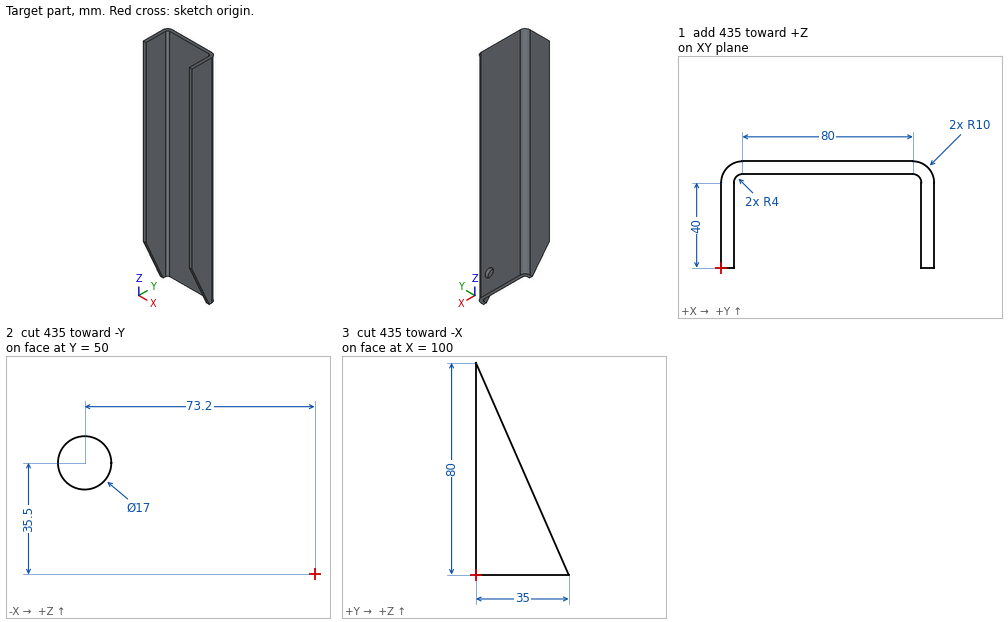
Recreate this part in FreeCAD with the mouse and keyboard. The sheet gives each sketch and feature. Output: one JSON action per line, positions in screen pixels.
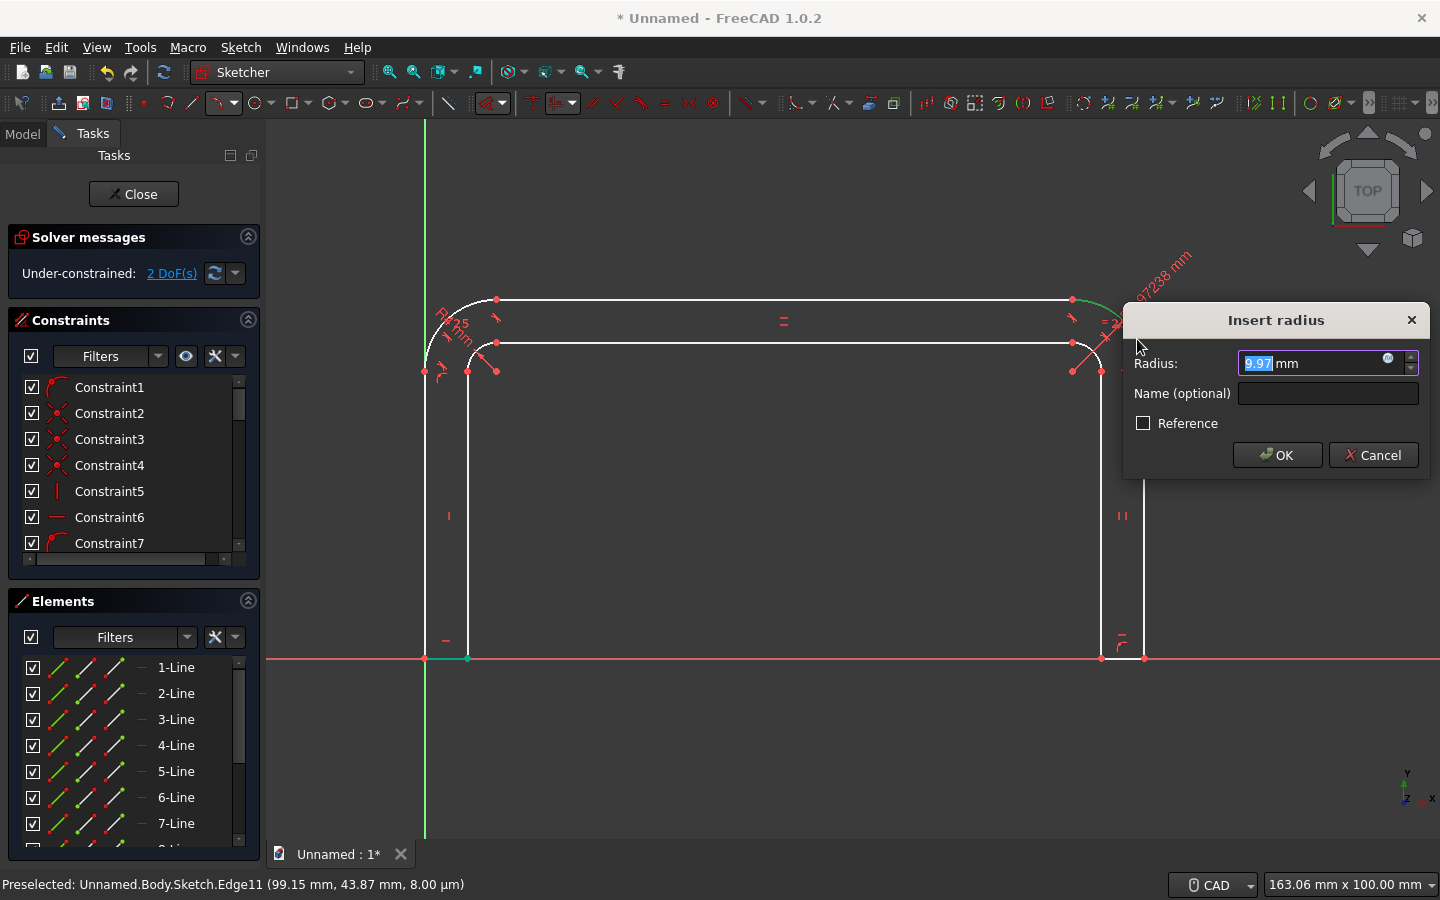
{"action": "type", "text": "10"}
{"action": "key", "text": "Return"}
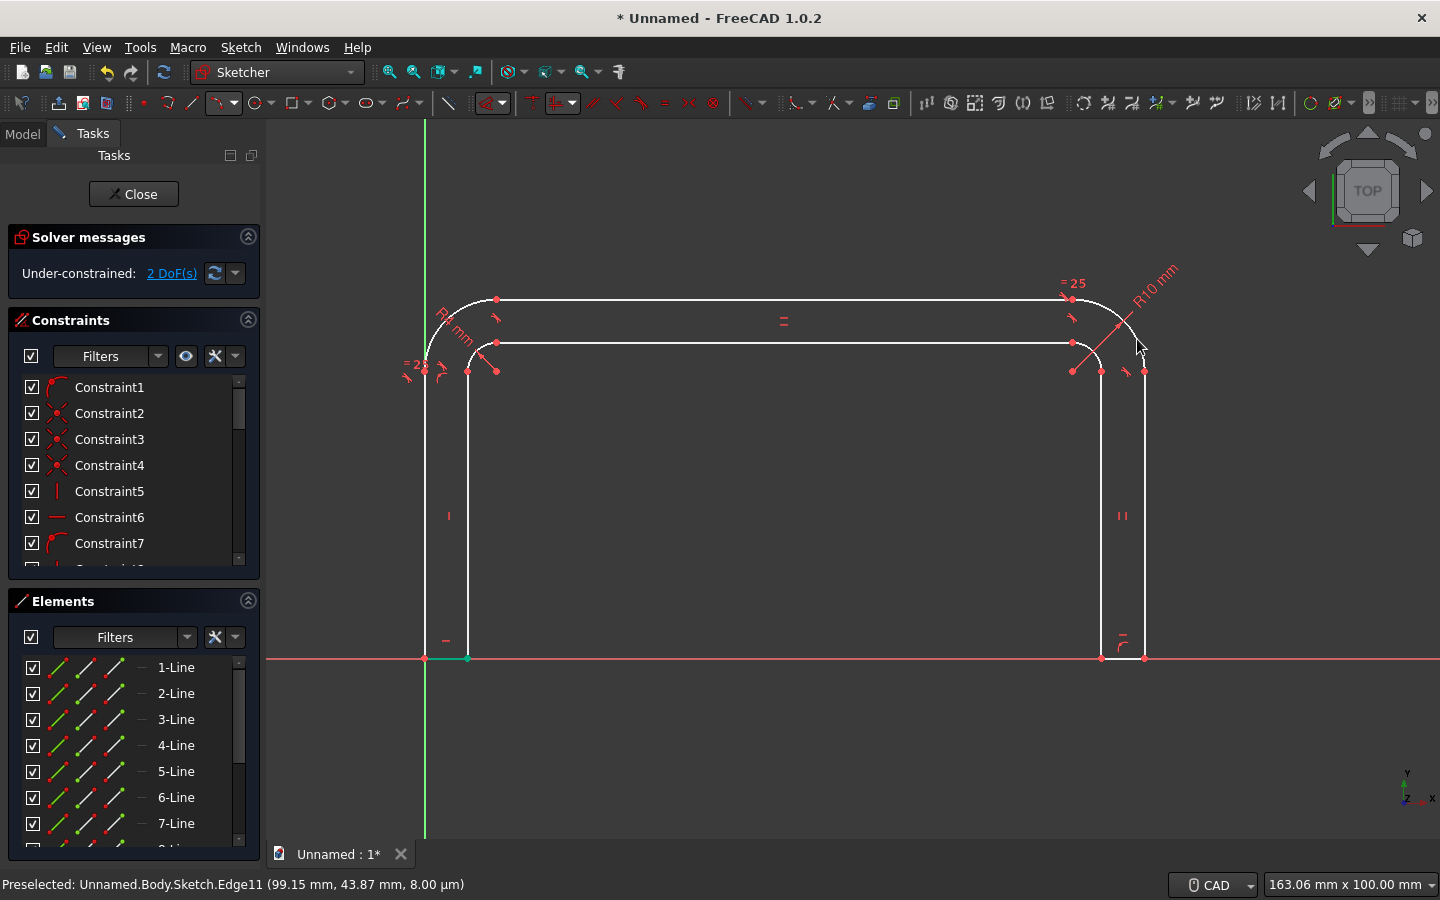
{"action": "left_click", "coordinate": [425, 458]}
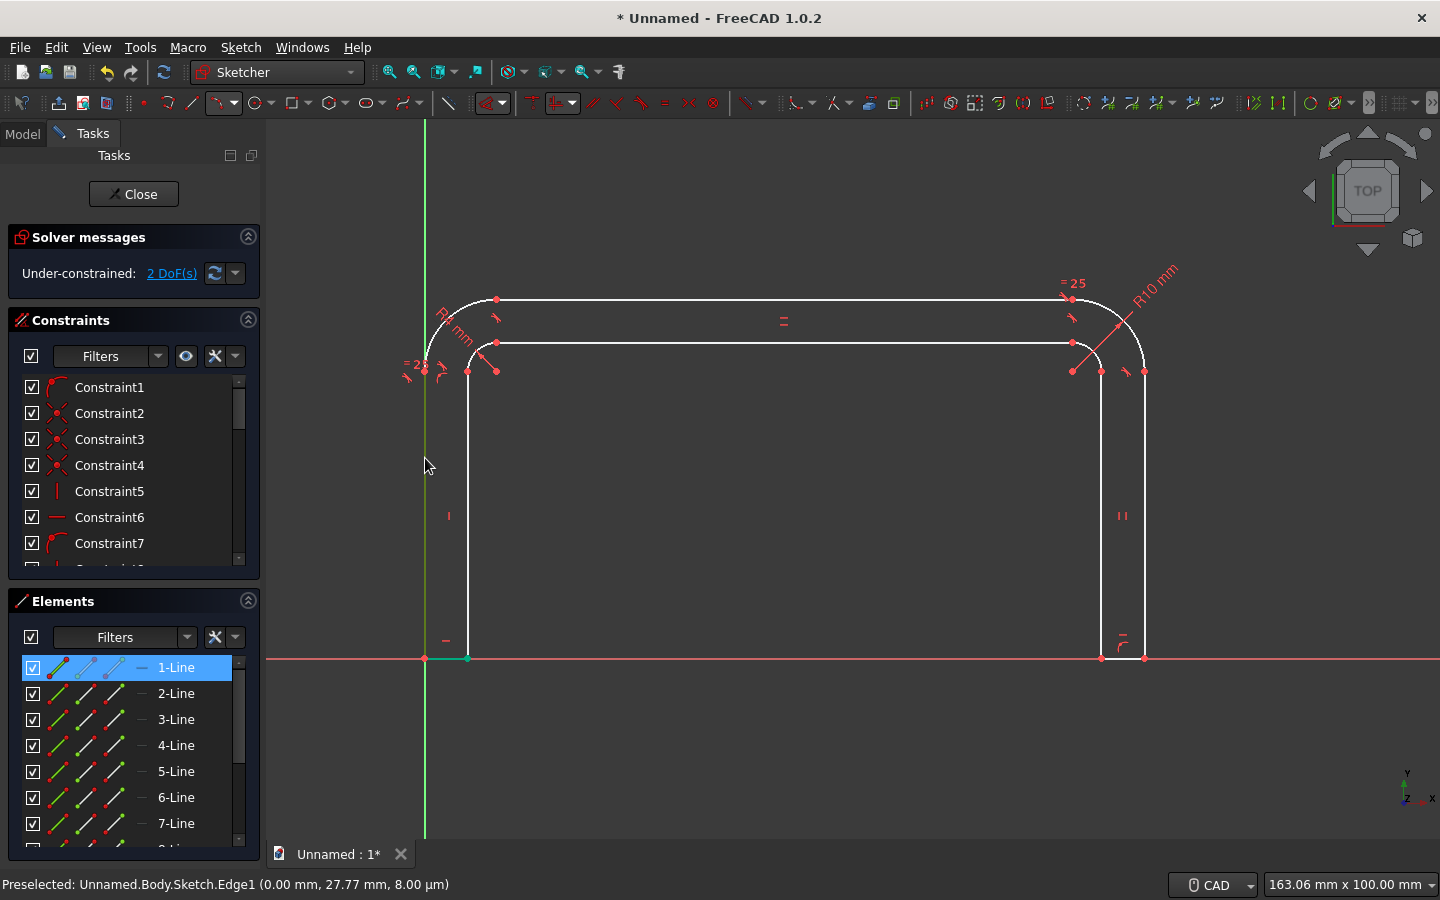
{"action": "left_click", "coordinate": [504, 104]}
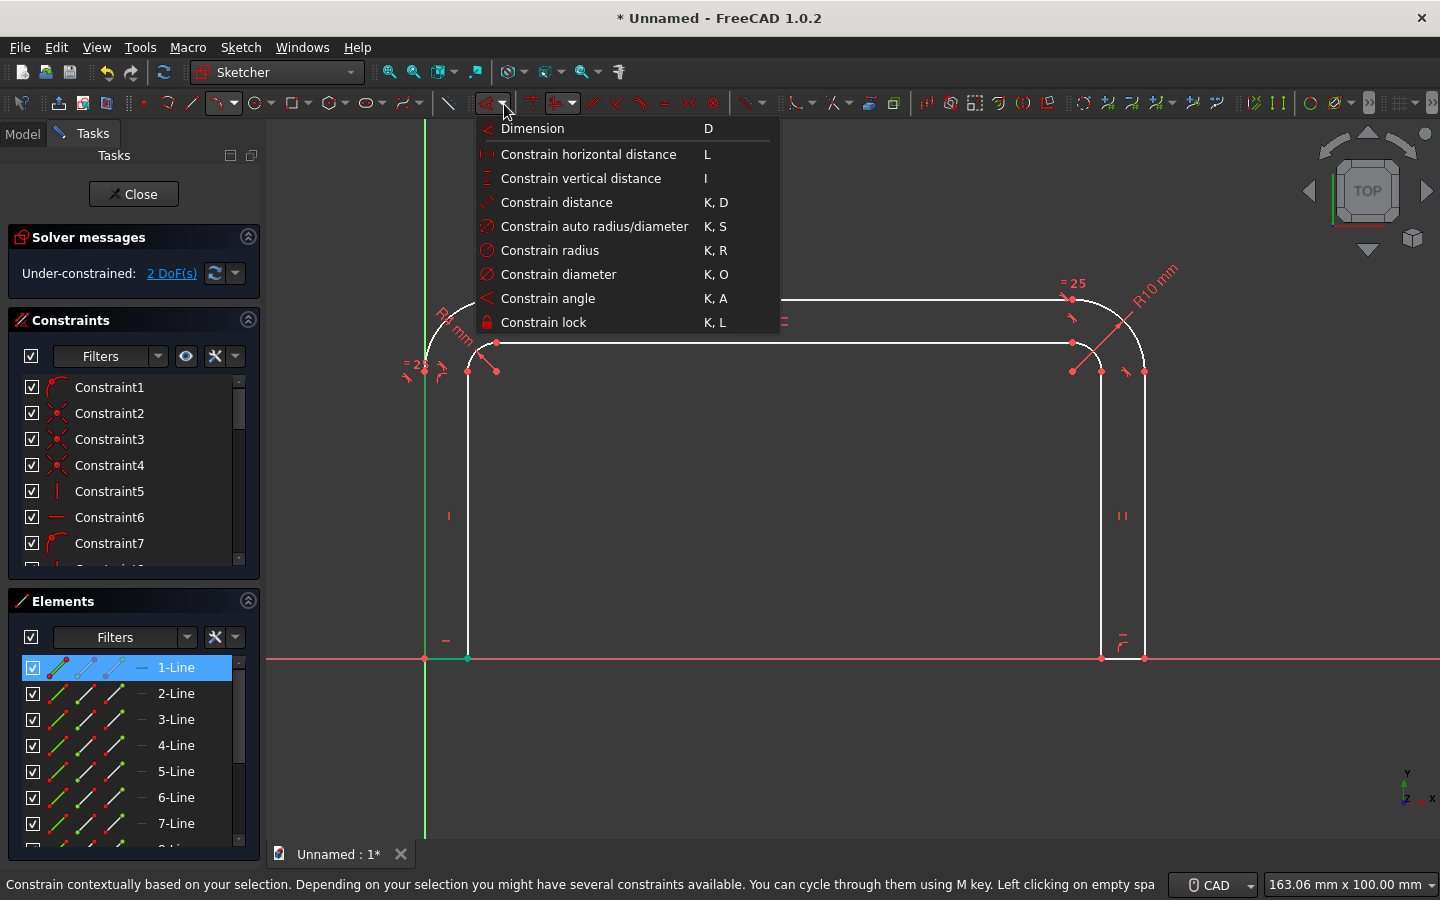
{"action": "left_click", "coordinate": [628, 178]}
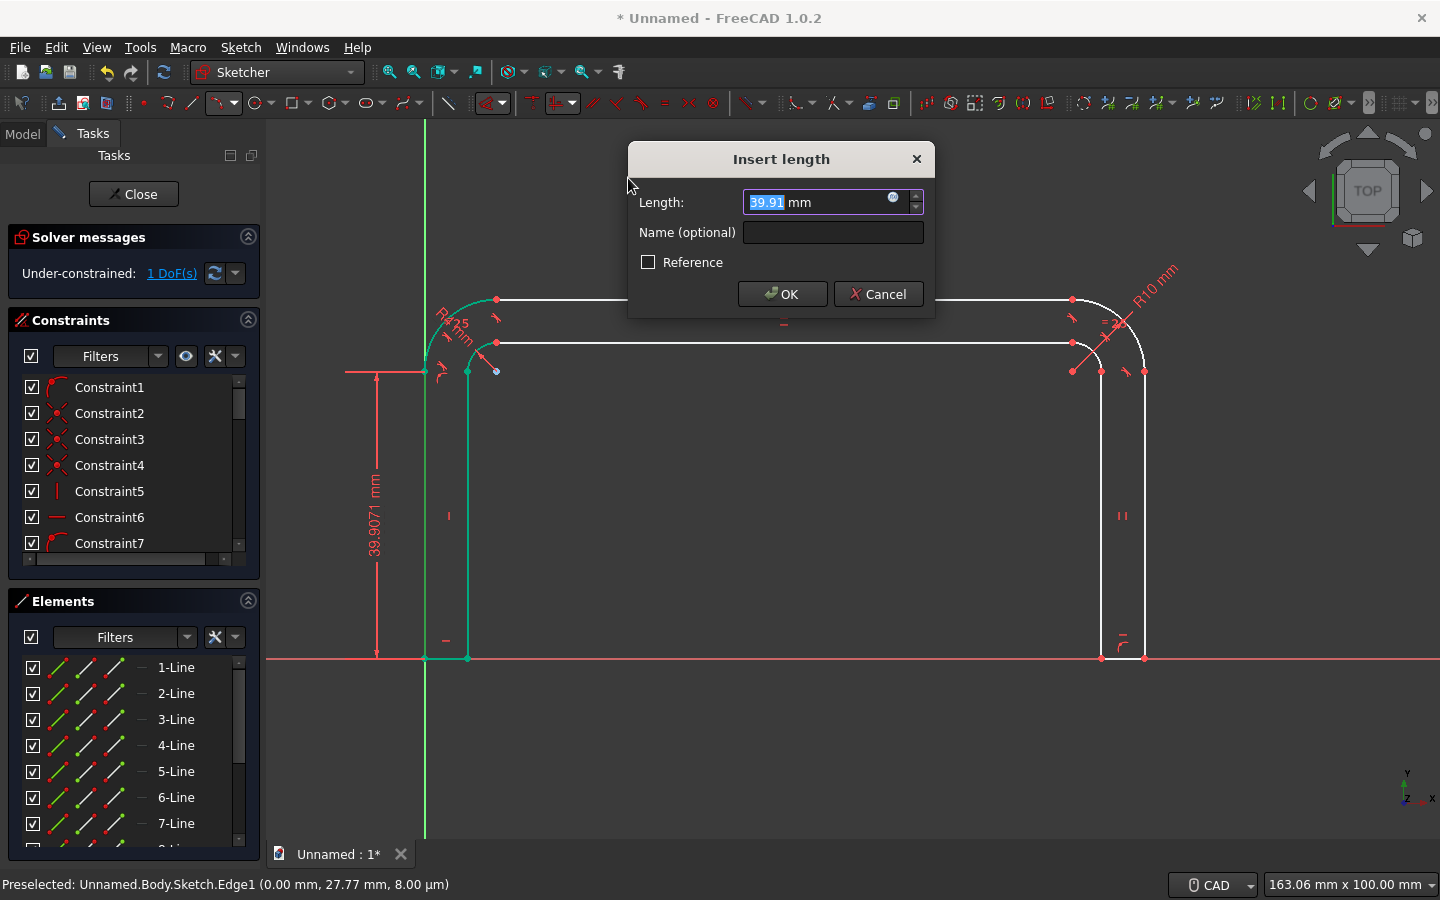
{"action": "type", "text": "40"}
{"action": "key", "text": "Return"}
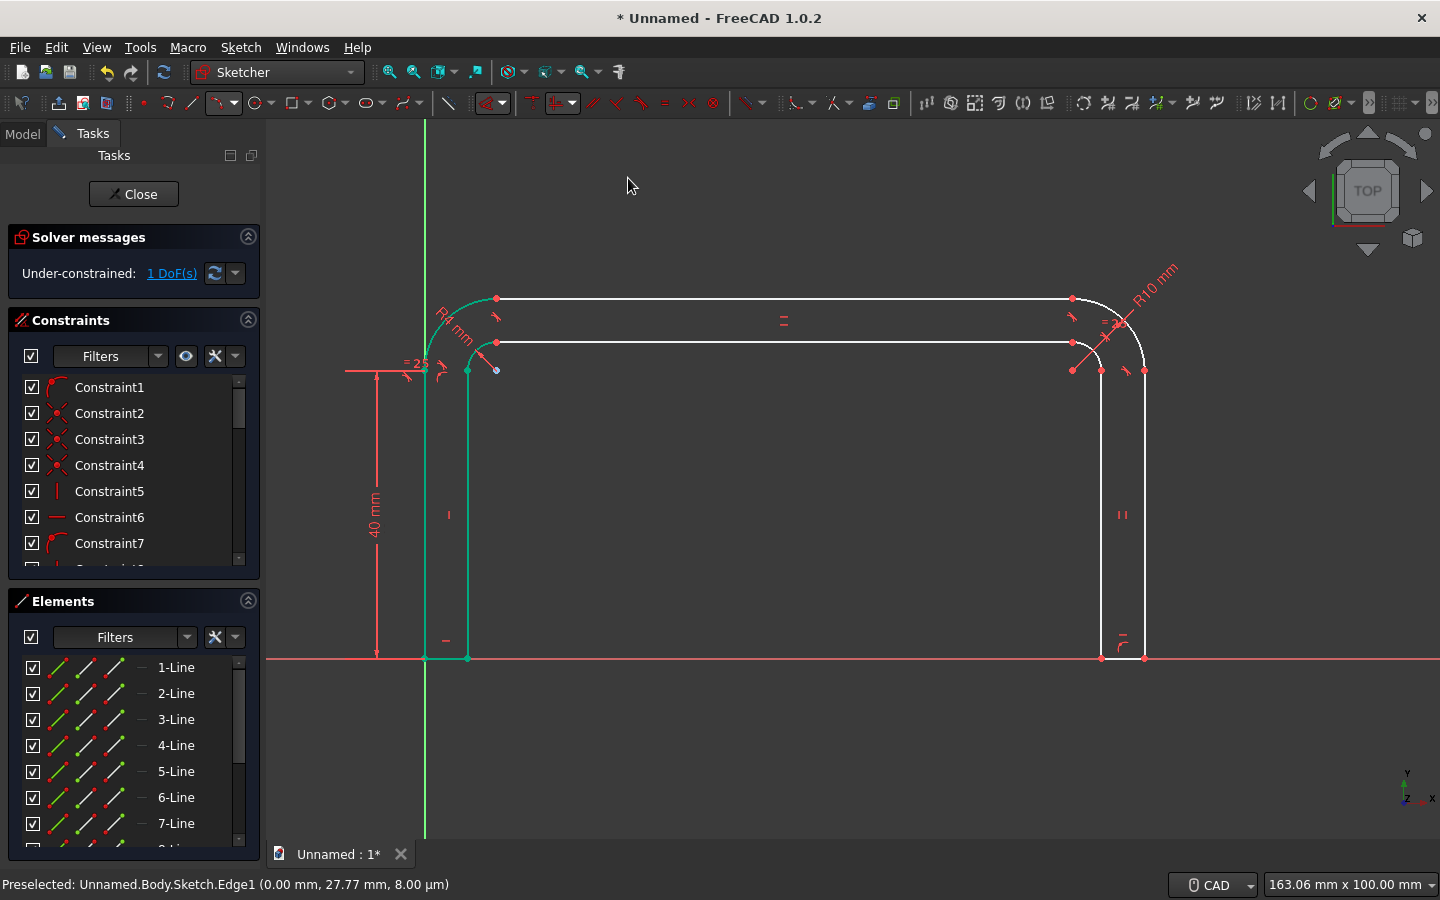
{"action": "left_click", "coordinate": [669, 342]}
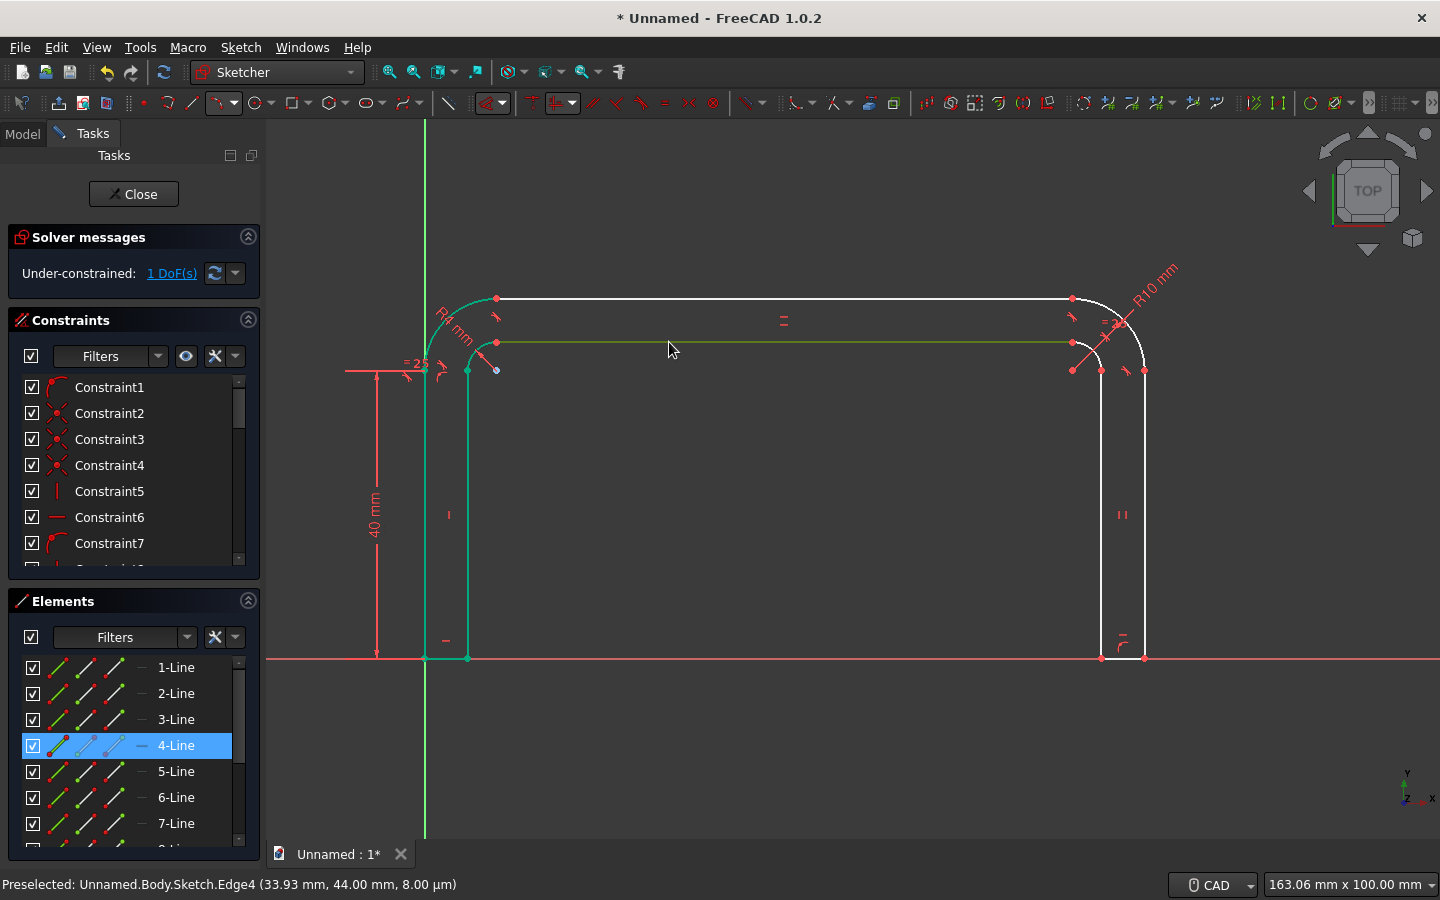
{"action": "left_click", "coordinate": [504, 104]}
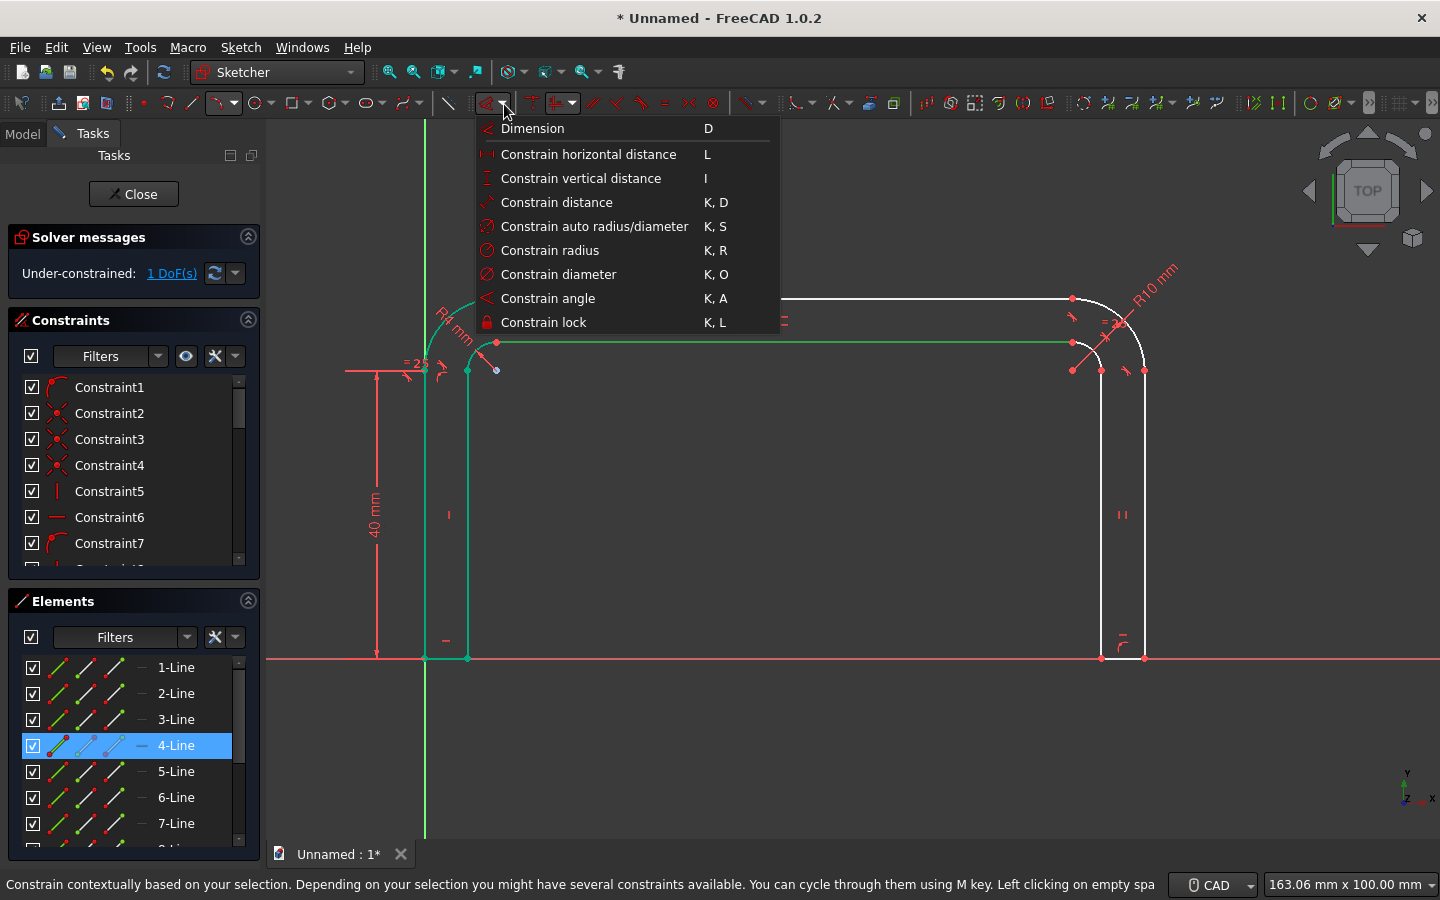
{"action": "left_click", "coordinate": [628, 154]}